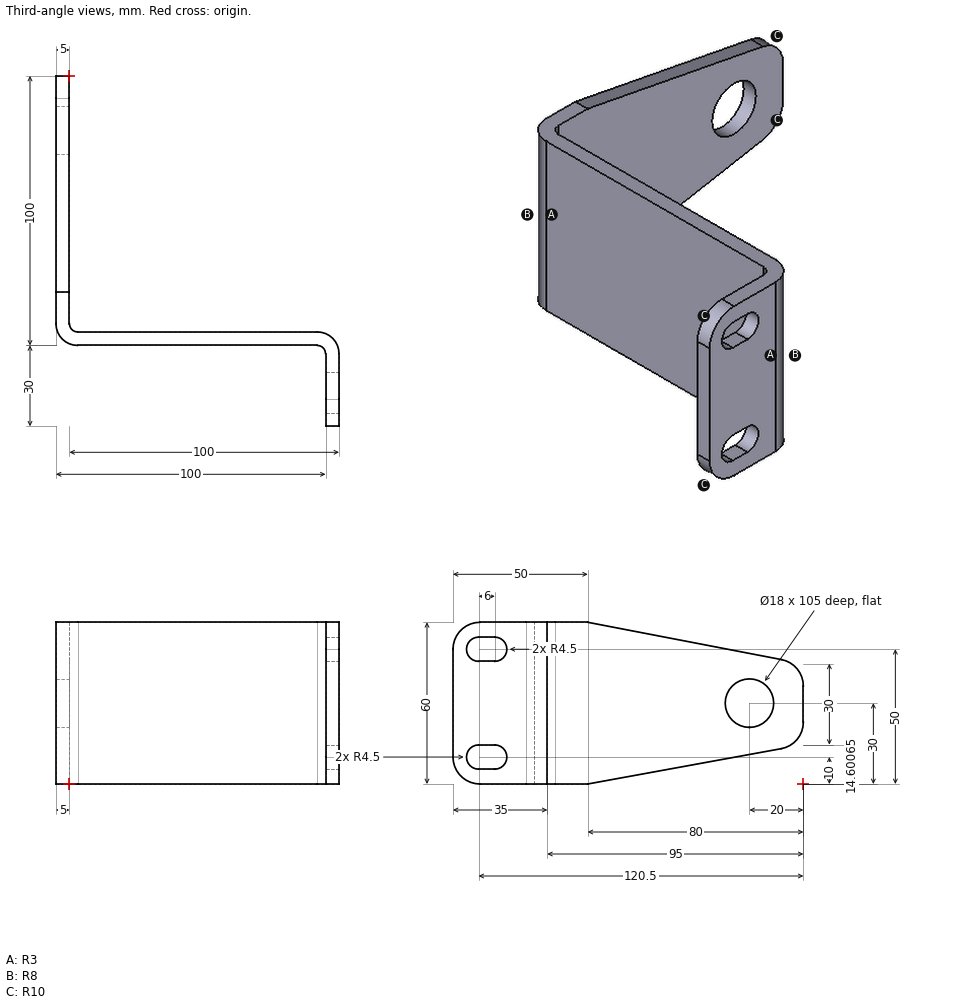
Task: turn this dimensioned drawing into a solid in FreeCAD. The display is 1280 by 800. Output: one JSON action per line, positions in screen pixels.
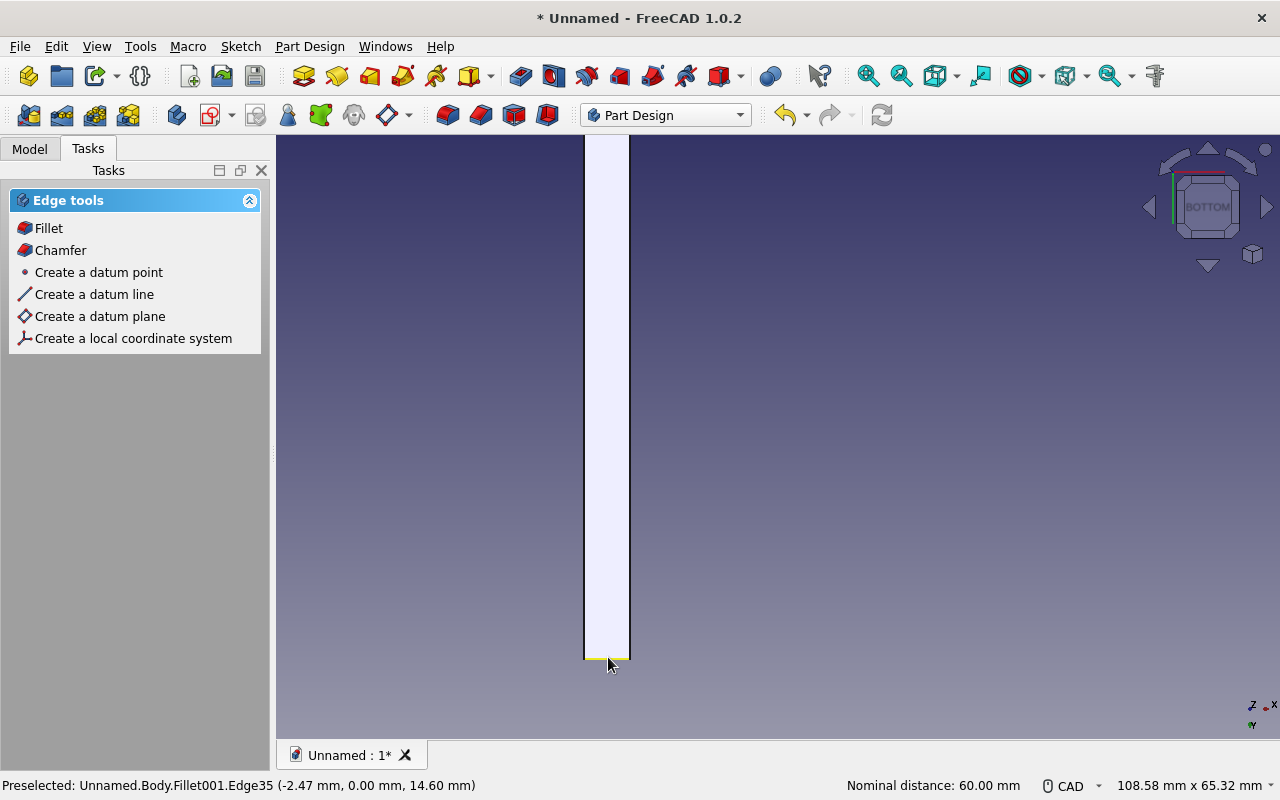
{"action": "left_click", "coordinate": [869, 76]}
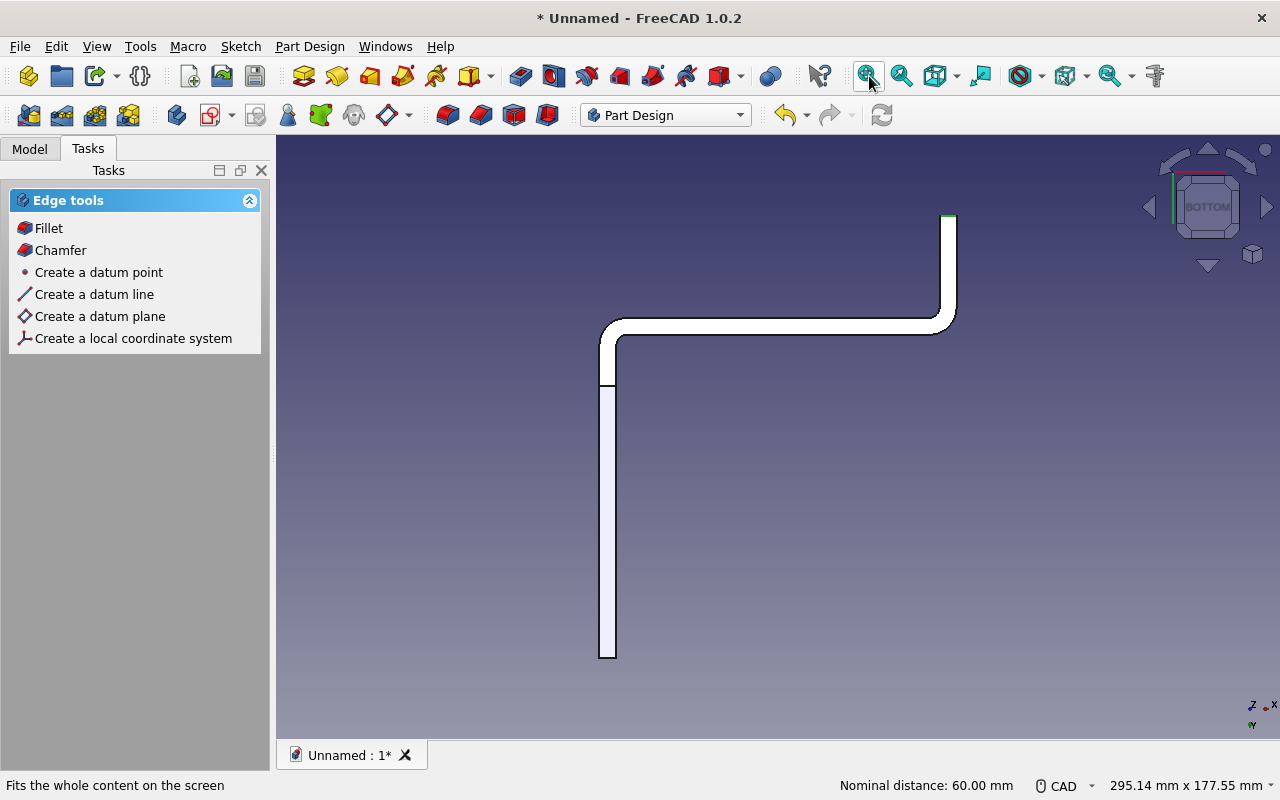
{"action": "key", "text": "4"}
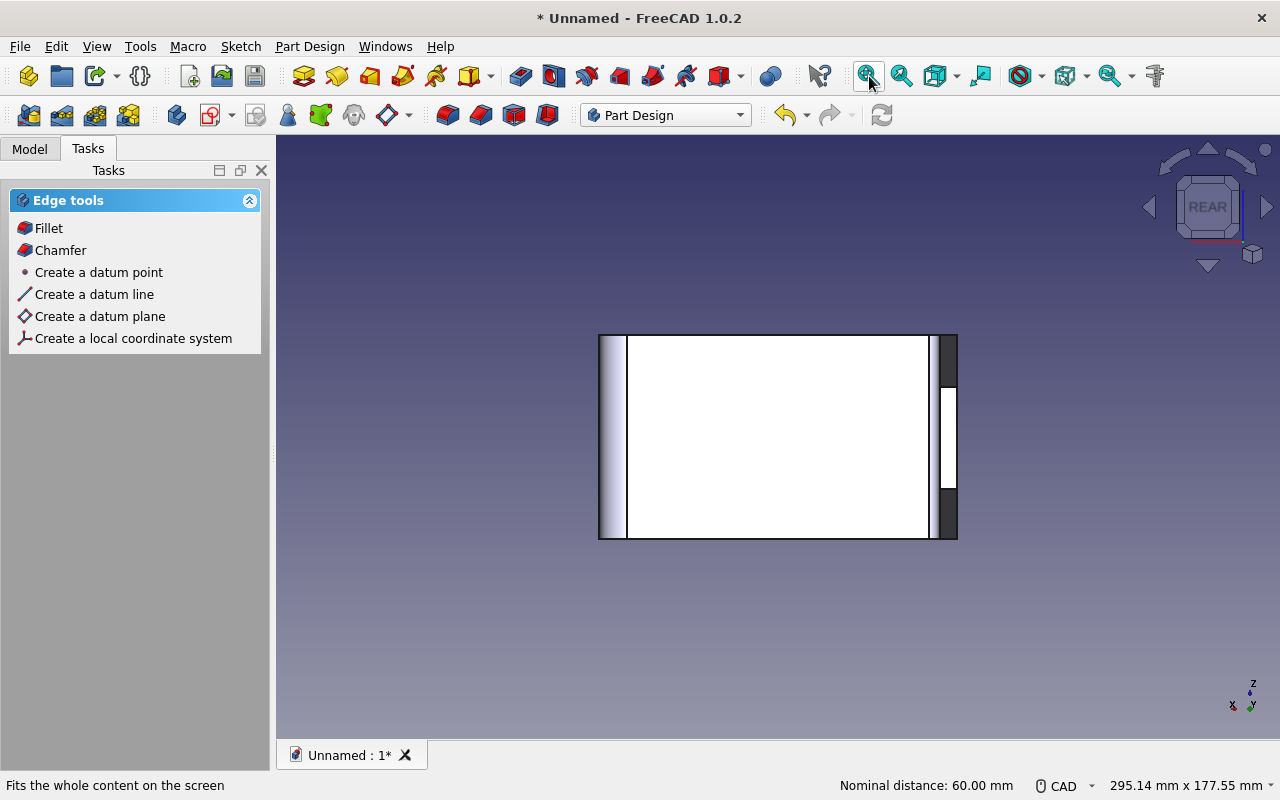
{"action": "left_click", "coordinate": [869, 76]}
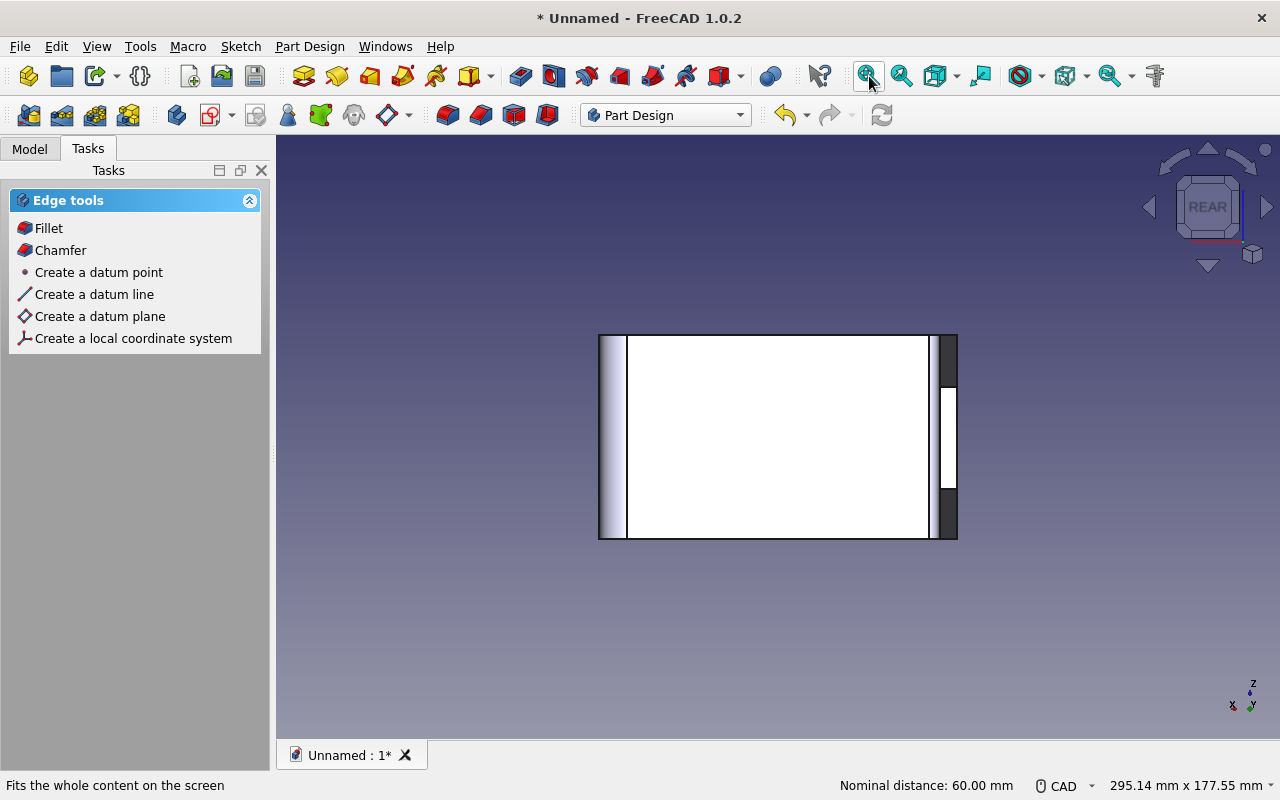
{"action": "left_click", "coordinate": [948, 386], "text": "ctrl"}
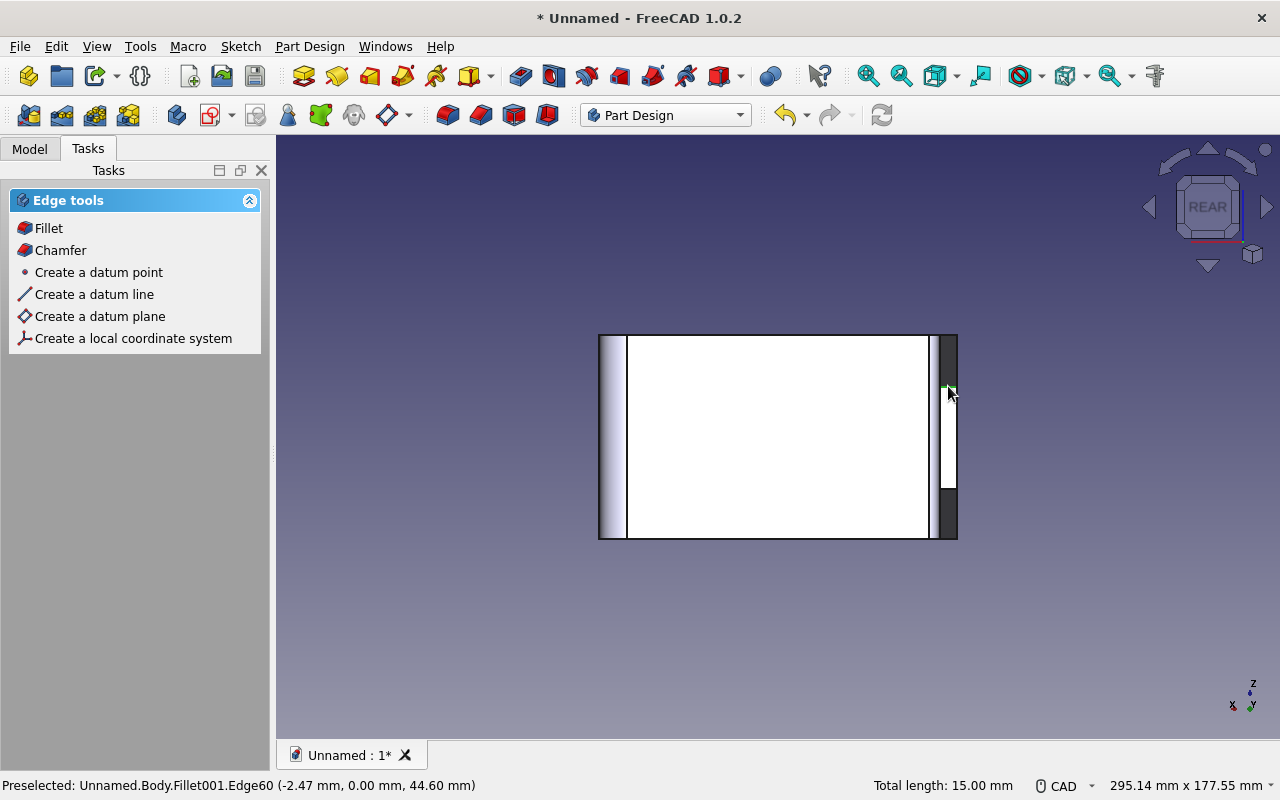
{"action": "scroll", "coordinate": [948, 488], "scroll_direction": "up", "scroll_amount": 5}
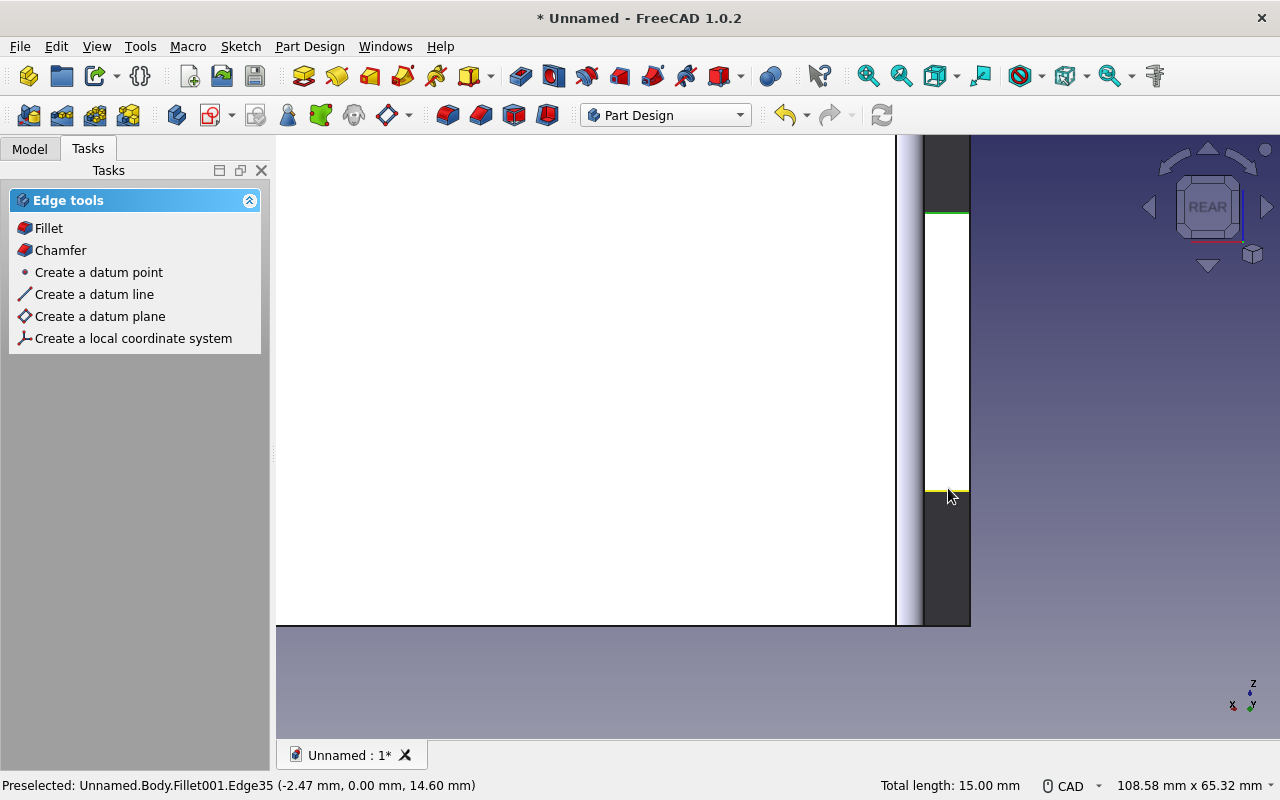
{"action": "left_click", "coordinate": [869, 76]}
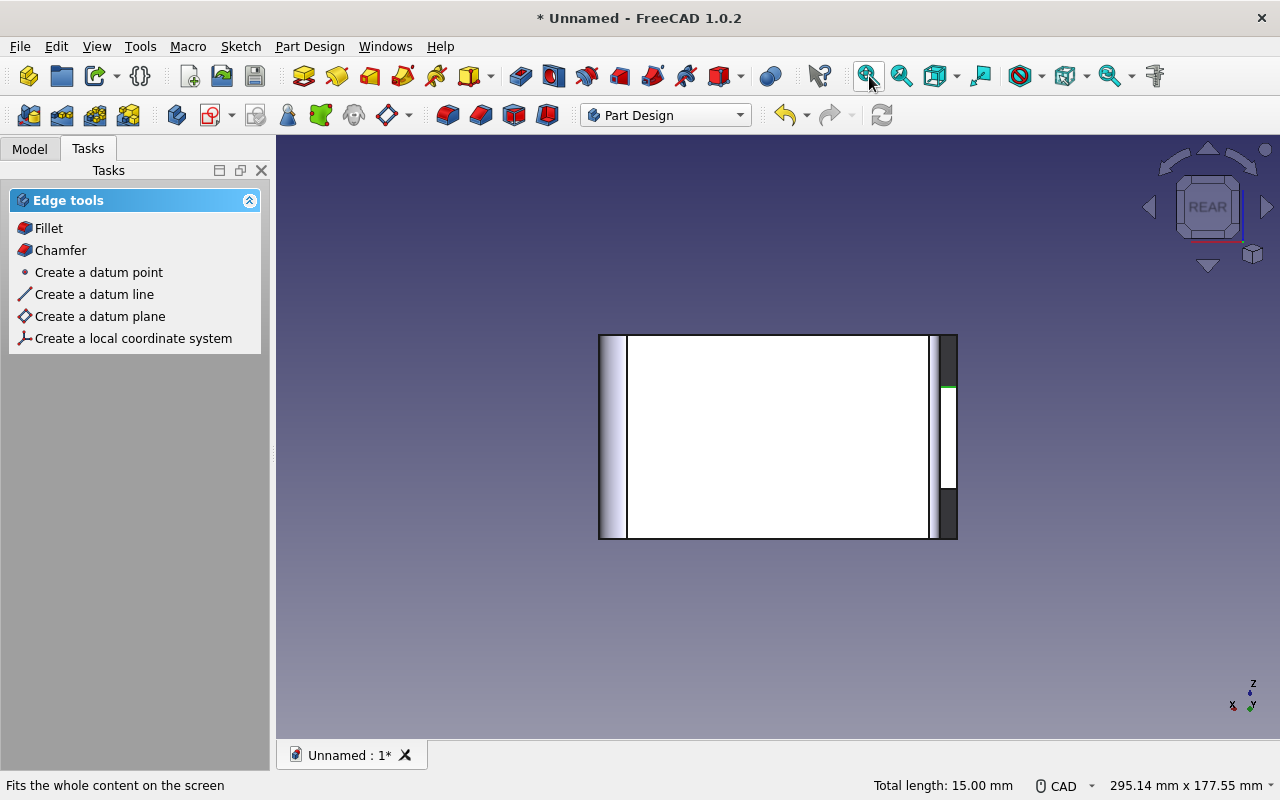
{"action": "key", "text": "6"}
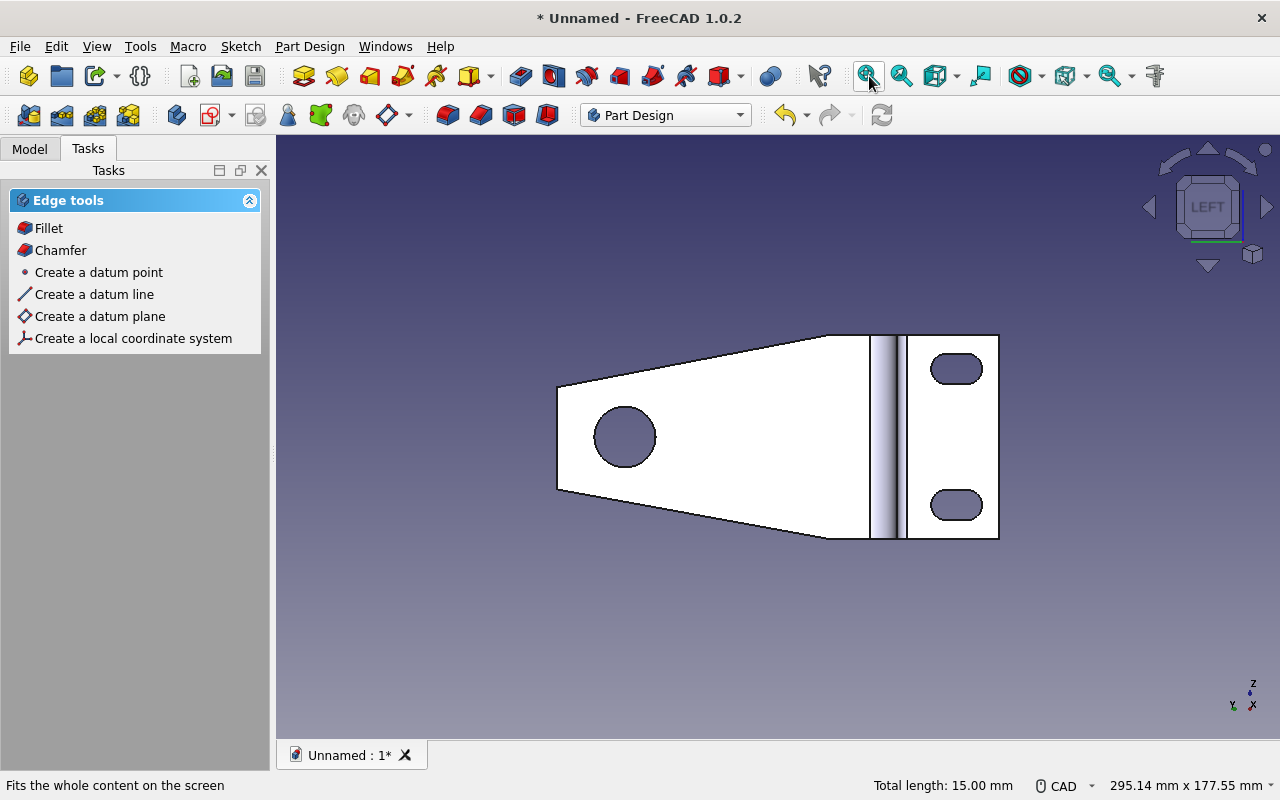
{"action": "left_click", "coordinate": [869, 76]}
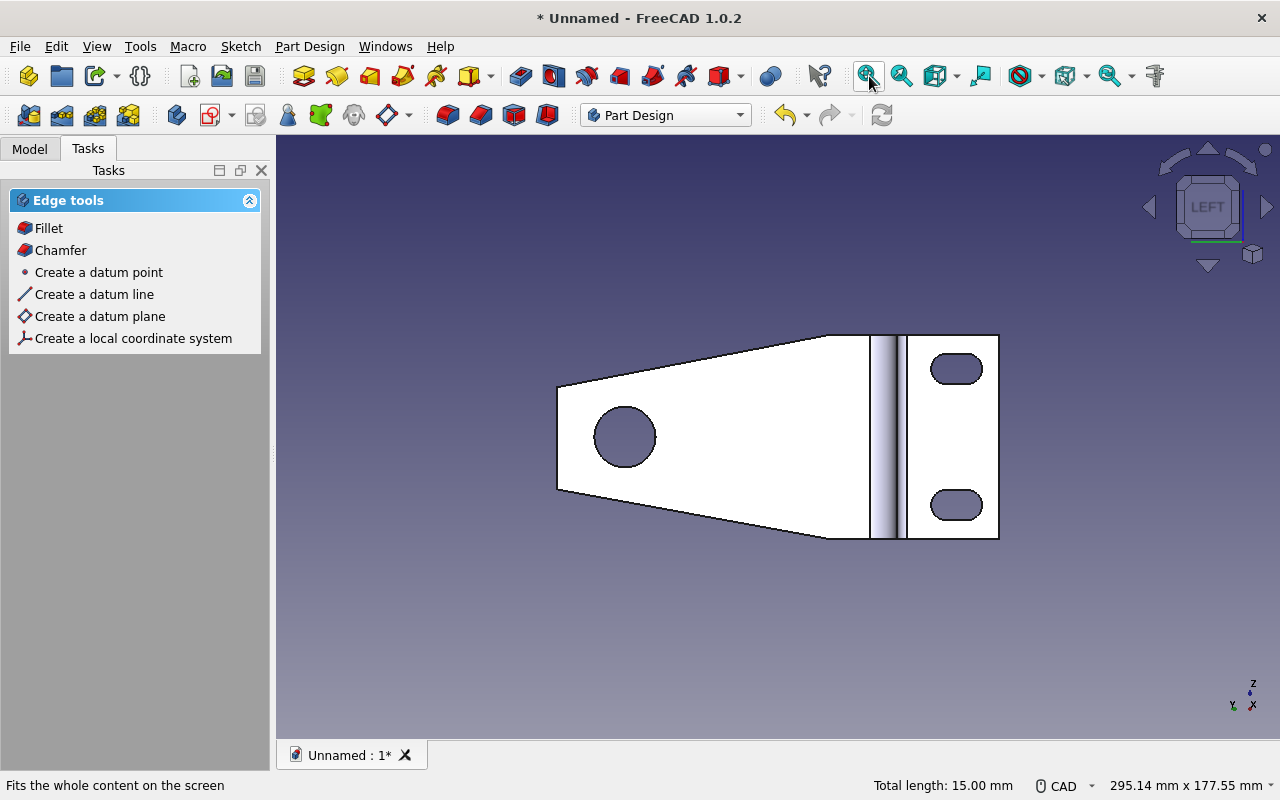
{"action": "scroll", "coordinate": [557, 488], "scroll_direction": "up", "scroll_amount": 5}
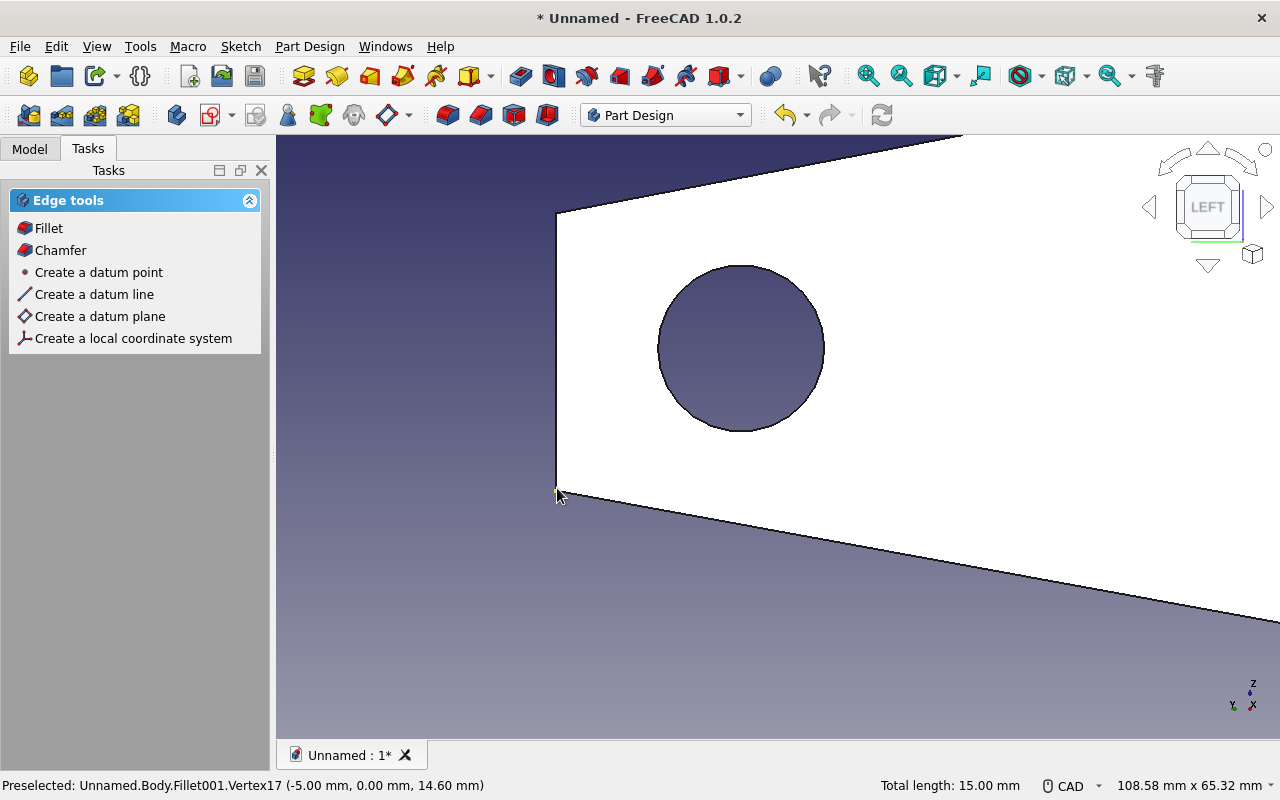
{"action": "left_click", "coordinate": [869, 76]}